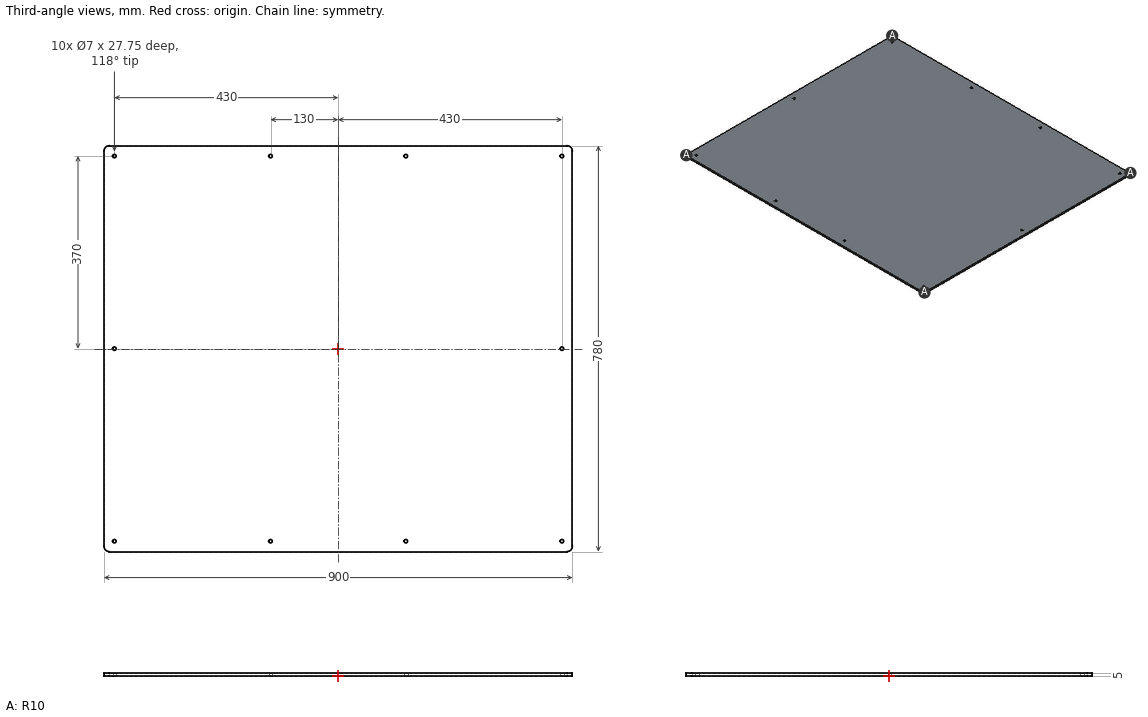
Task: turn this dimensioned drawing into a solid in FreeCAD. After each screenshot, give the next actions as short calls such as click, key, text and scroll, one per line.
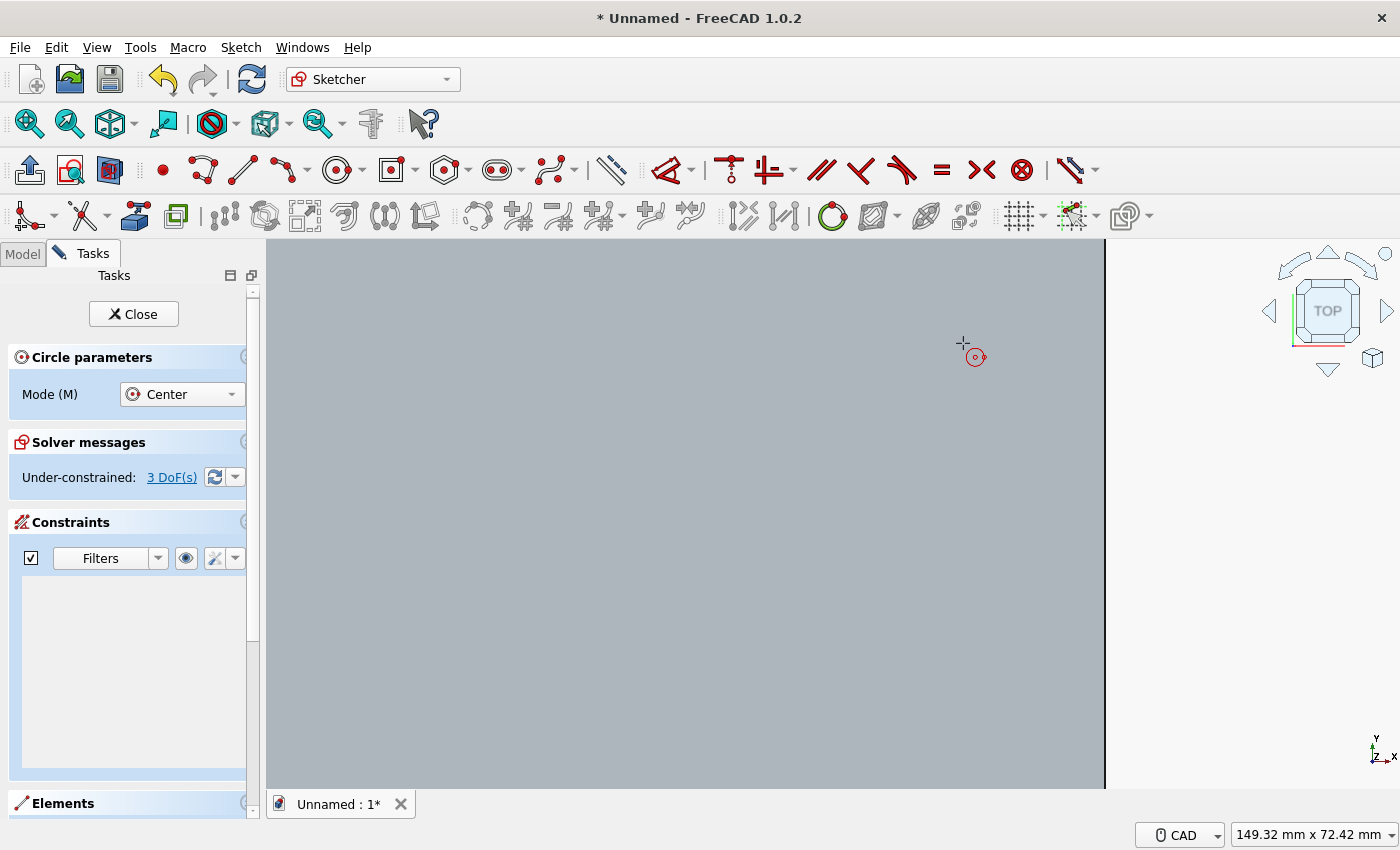
scroll(964, 343, down, 14)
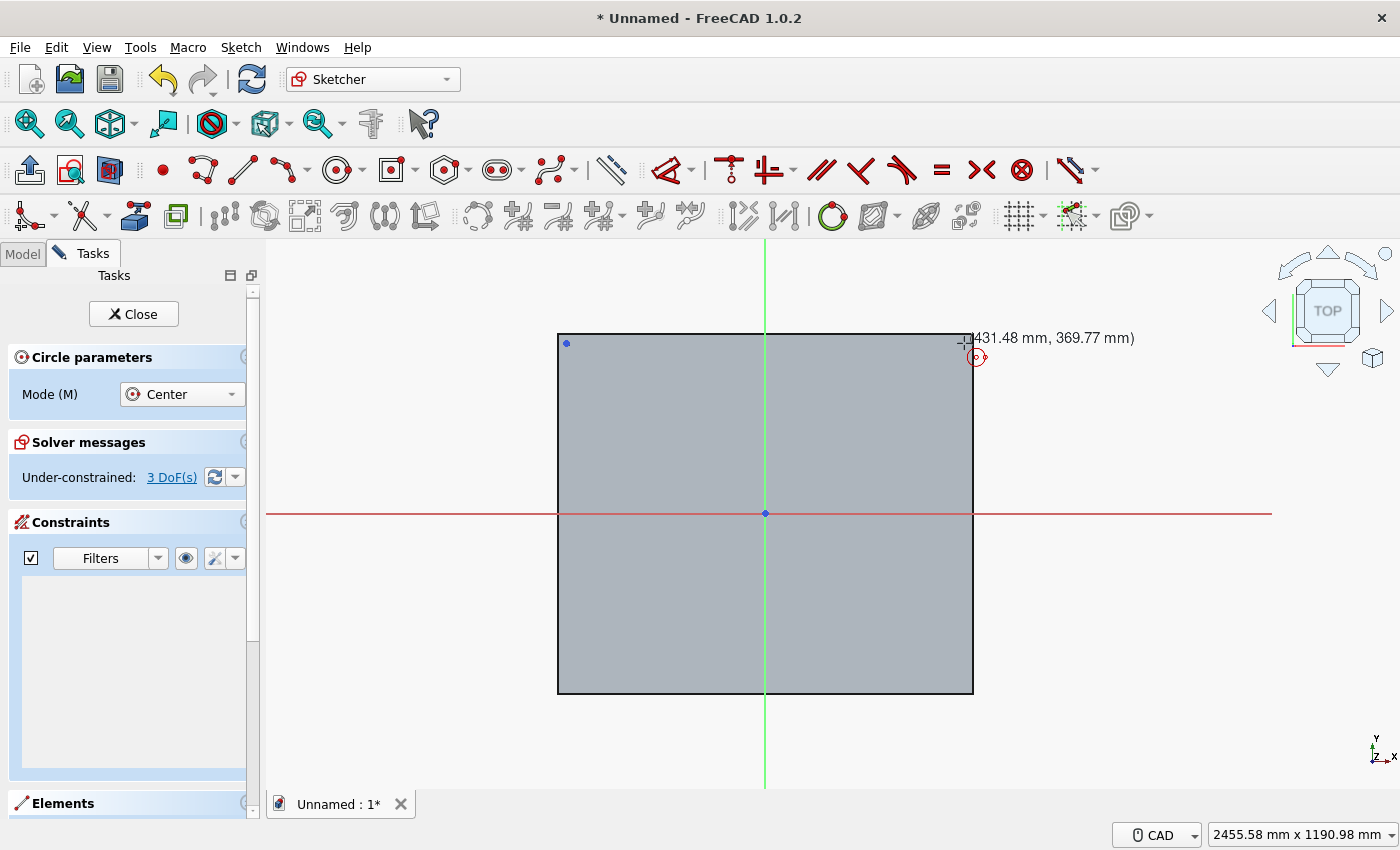
click(964, 343)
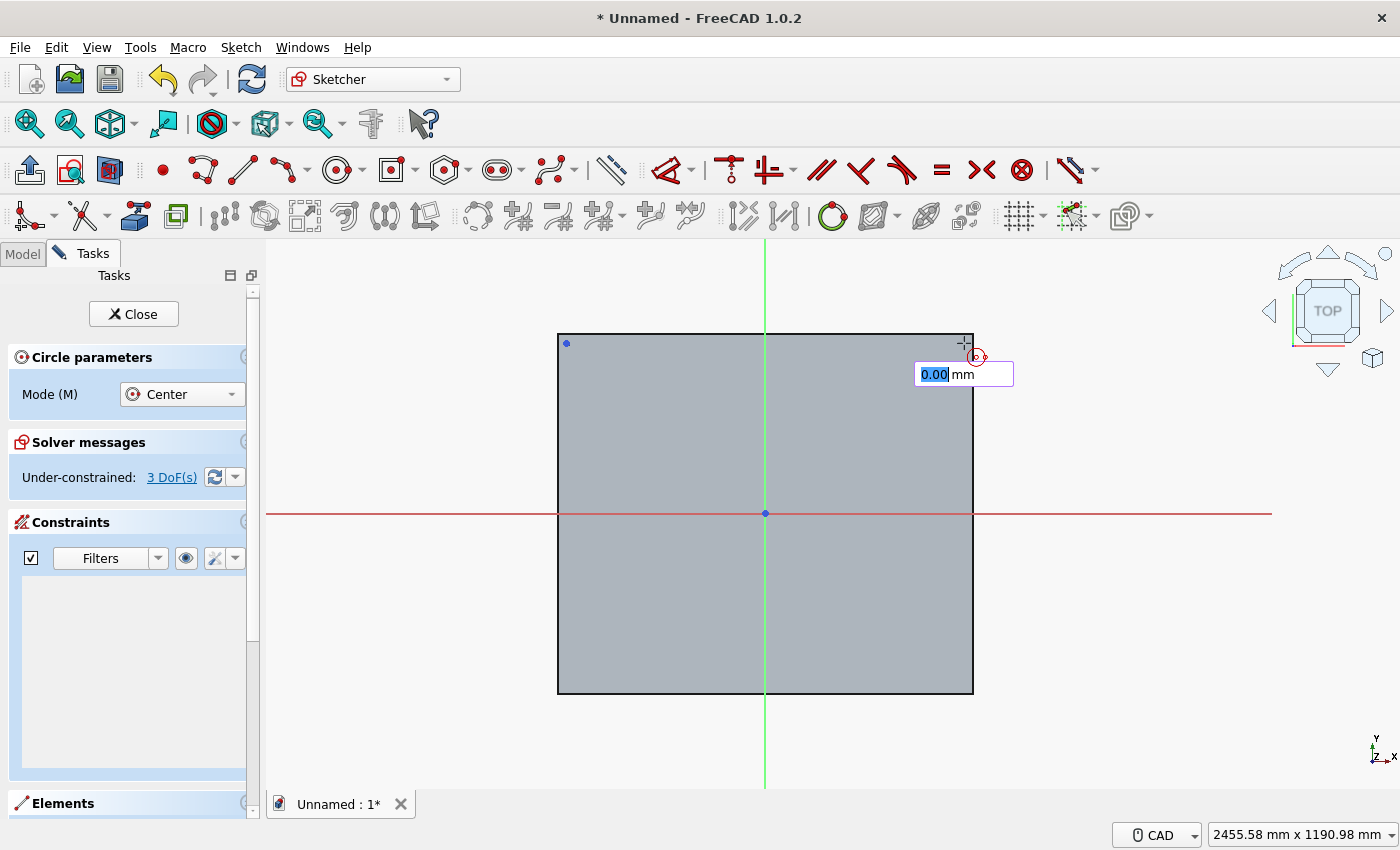
scroll(965, 342, up, 12)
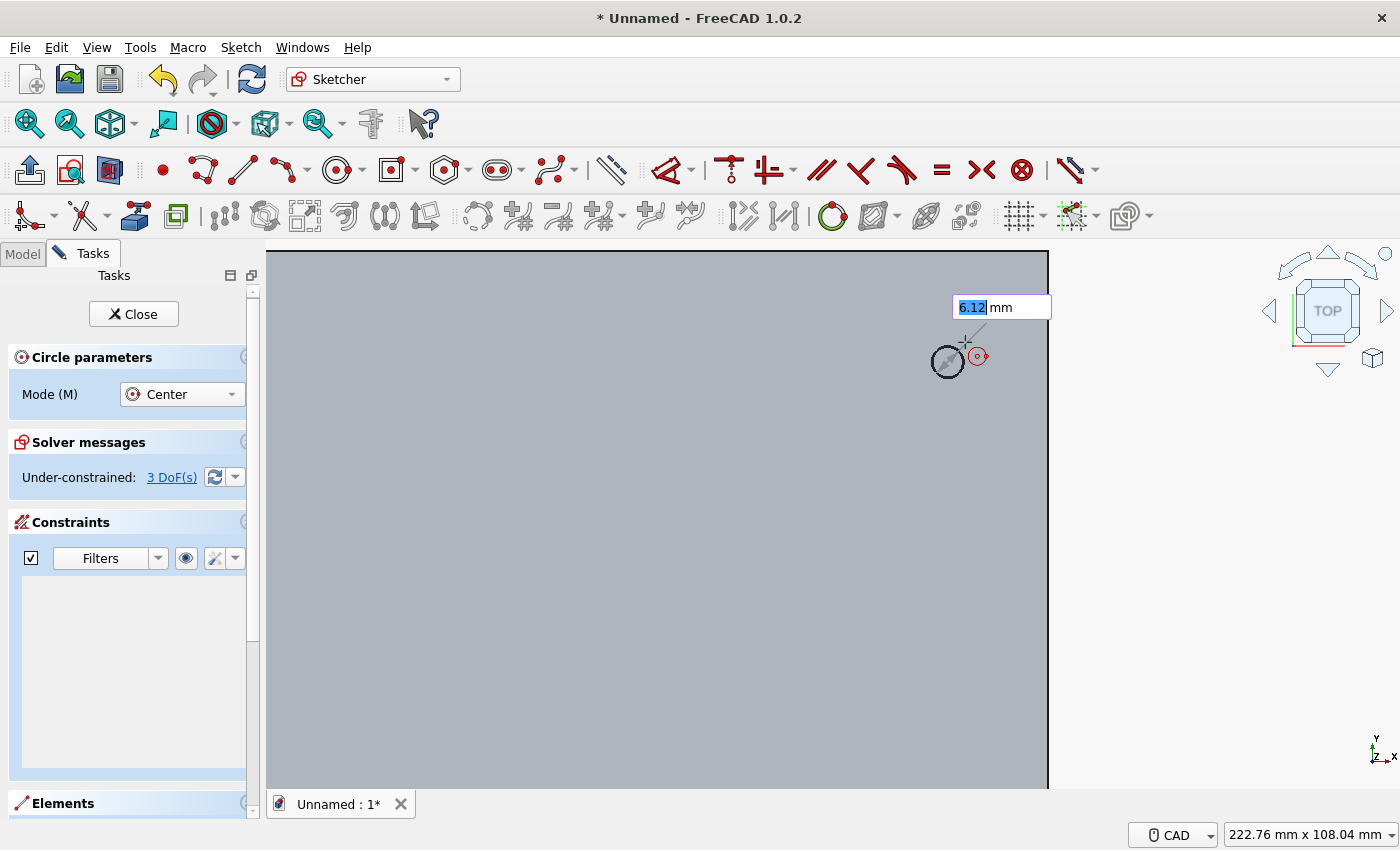
click(959, 340)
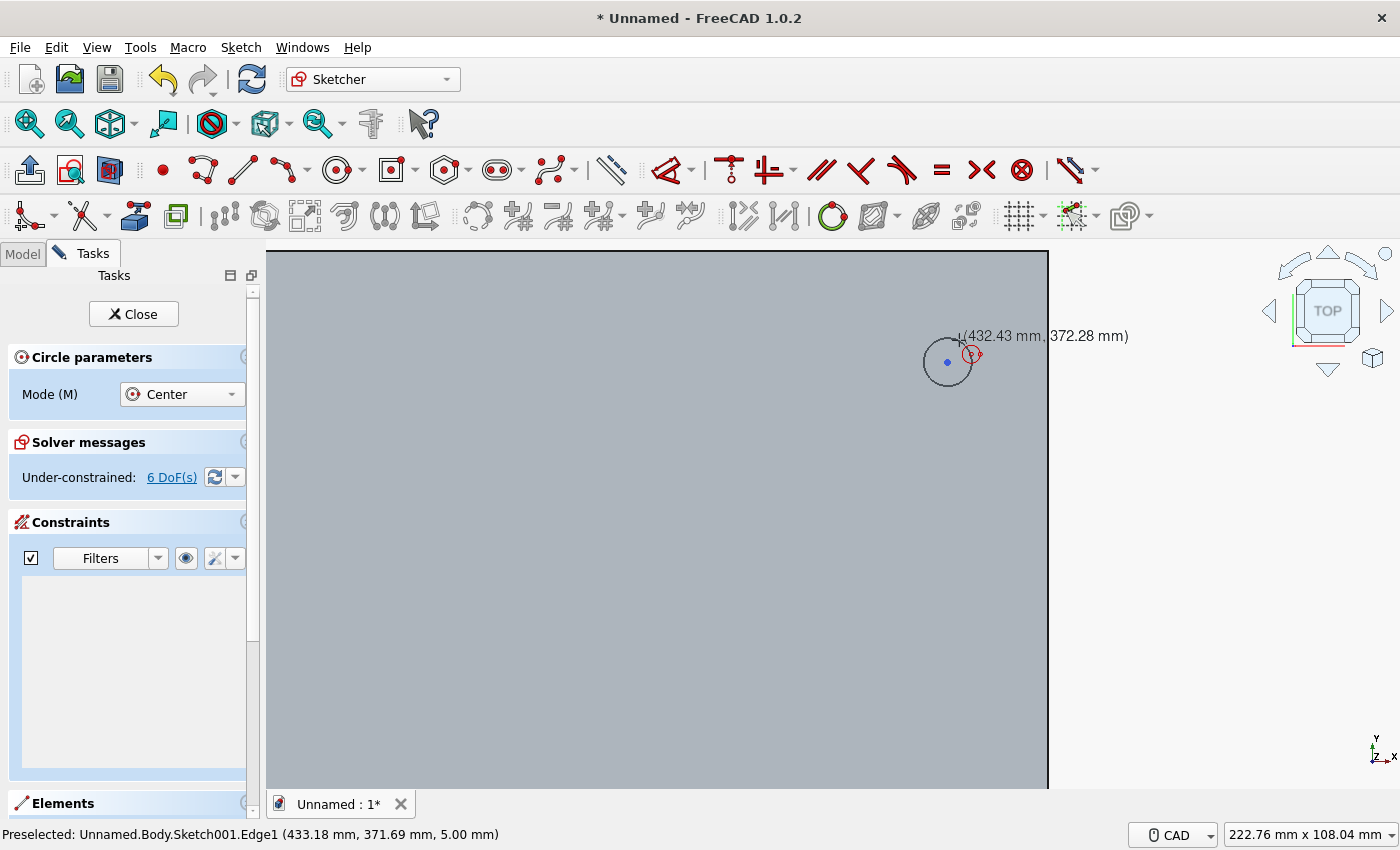
scroll(965, 342, down, 12)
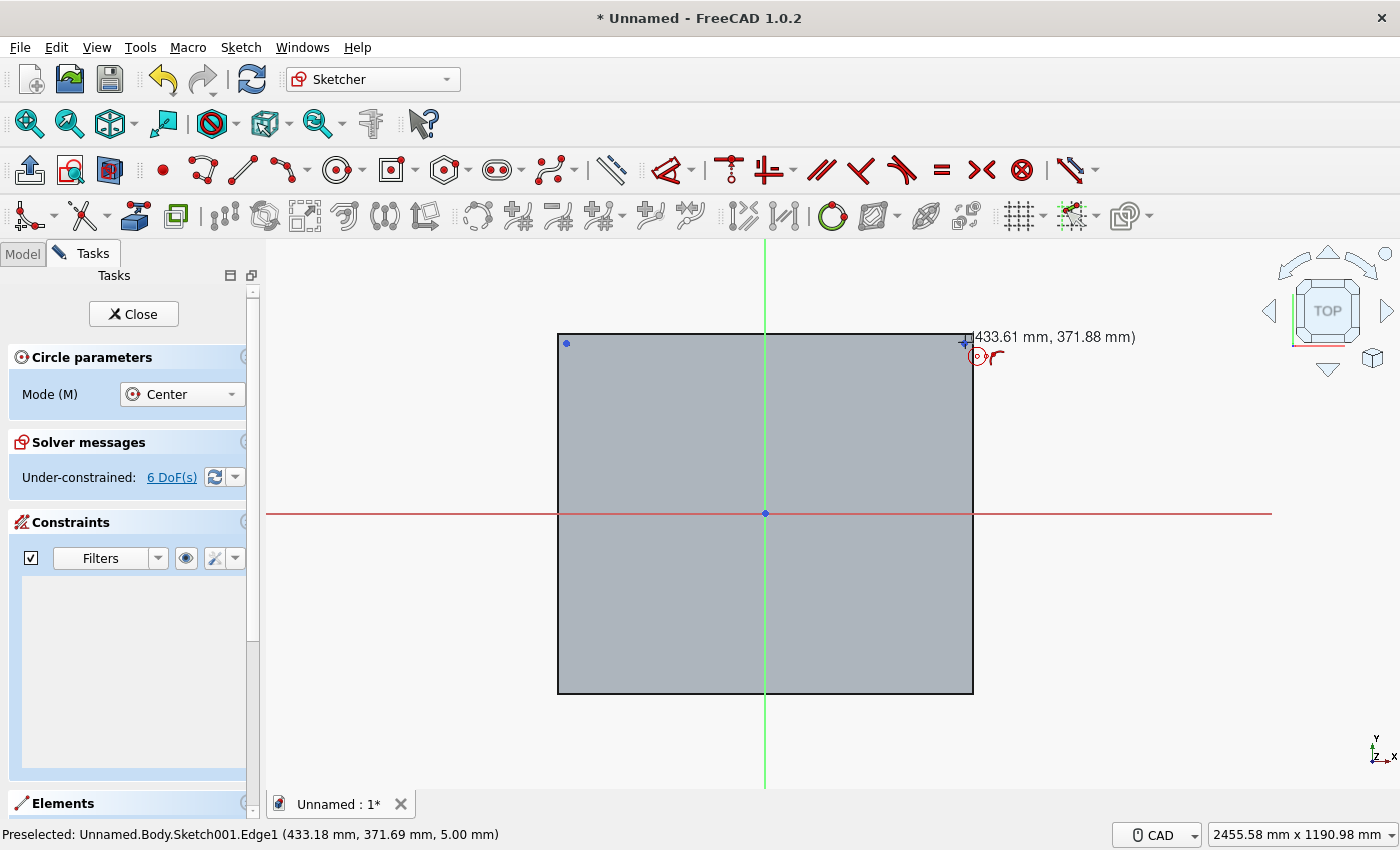
scroll(964, 685, up, 14)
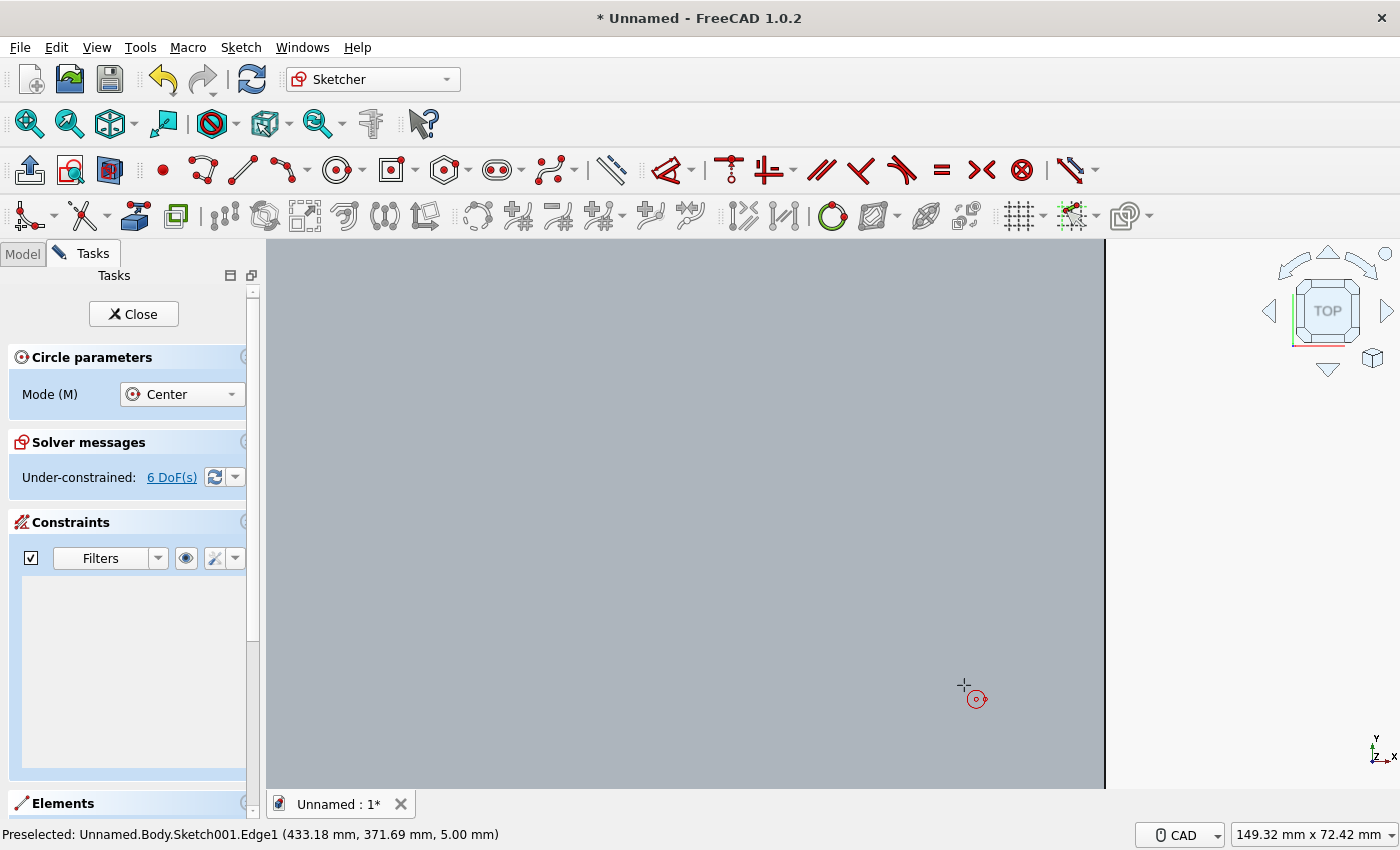
scroll(964, 686, down, 14)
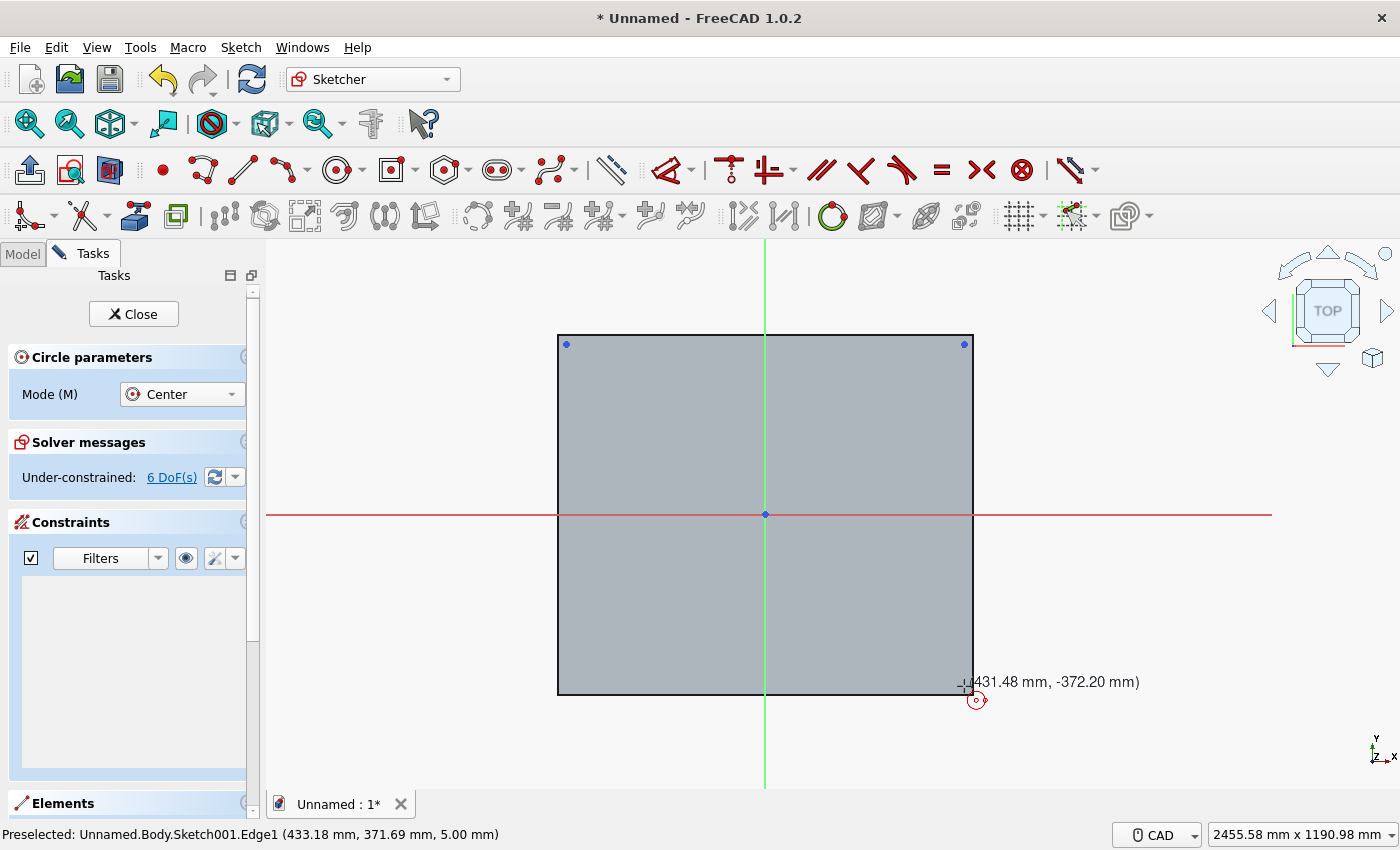
click(964, 686)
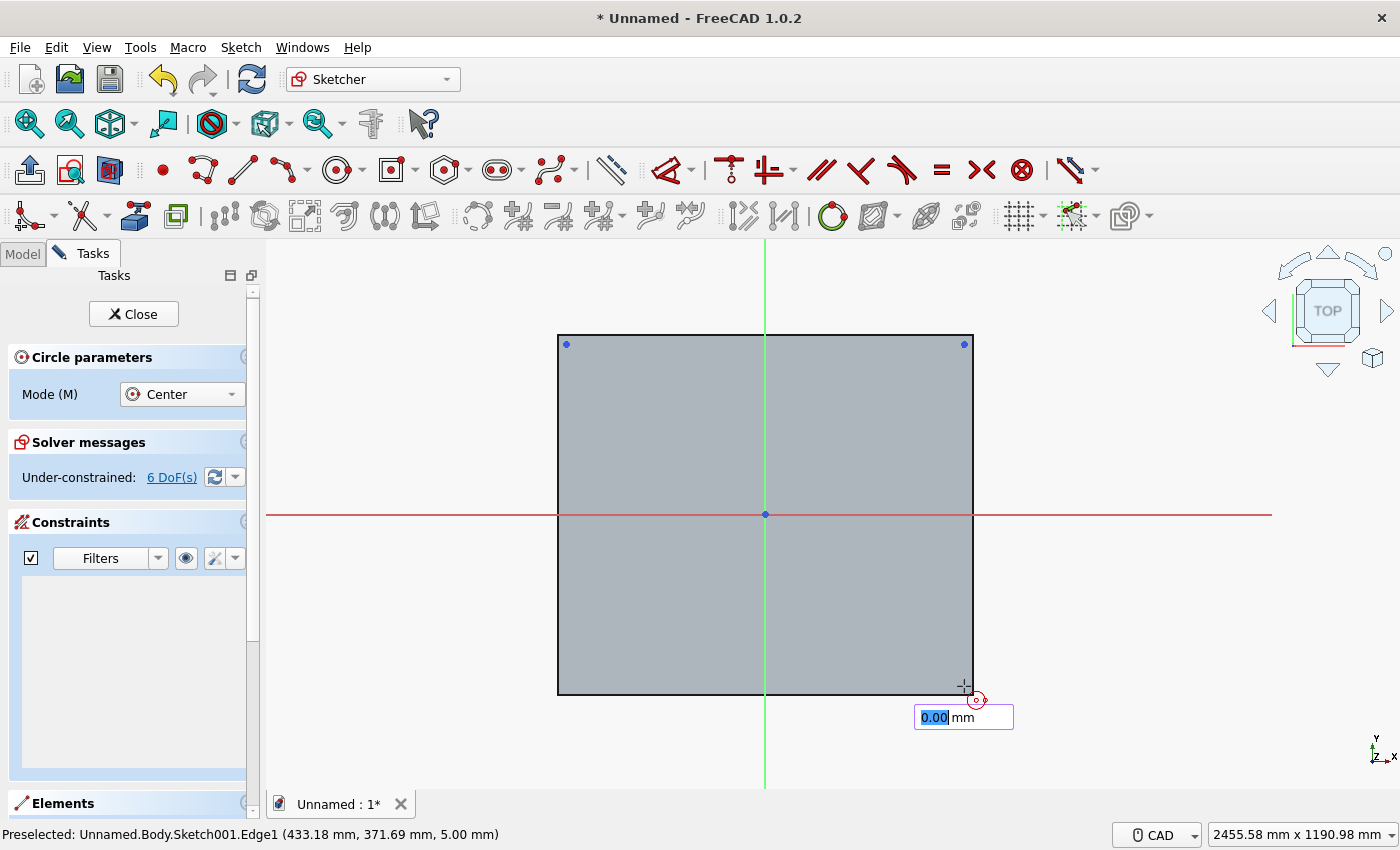
scroll(965, 685, up, 12)